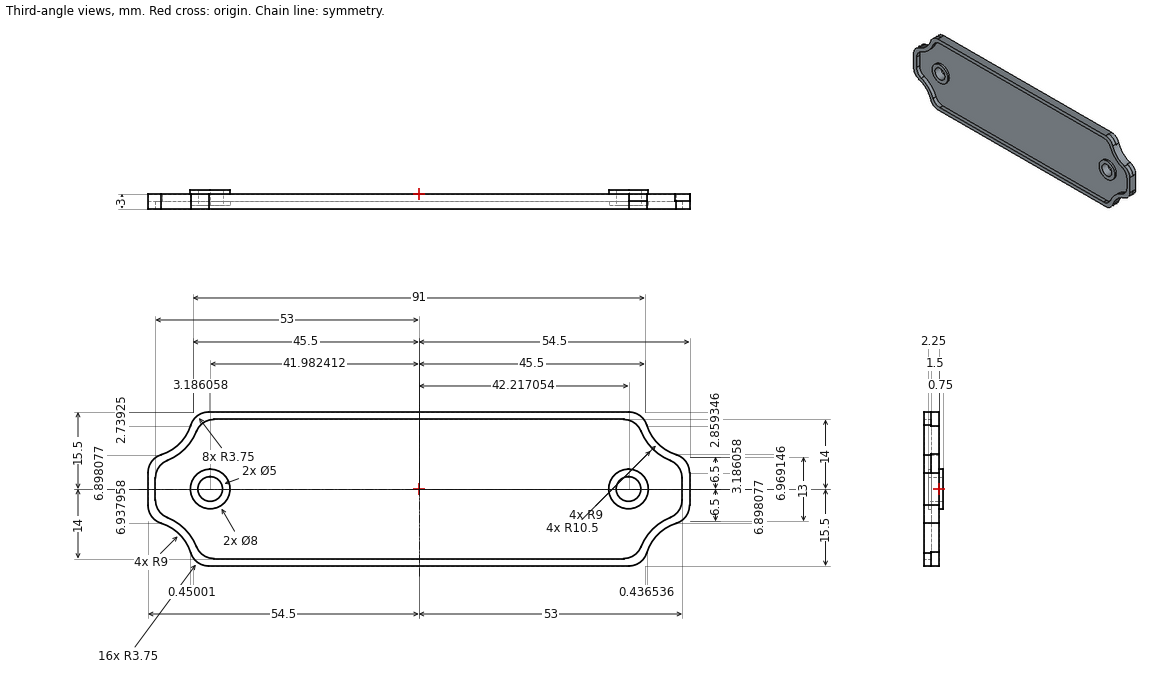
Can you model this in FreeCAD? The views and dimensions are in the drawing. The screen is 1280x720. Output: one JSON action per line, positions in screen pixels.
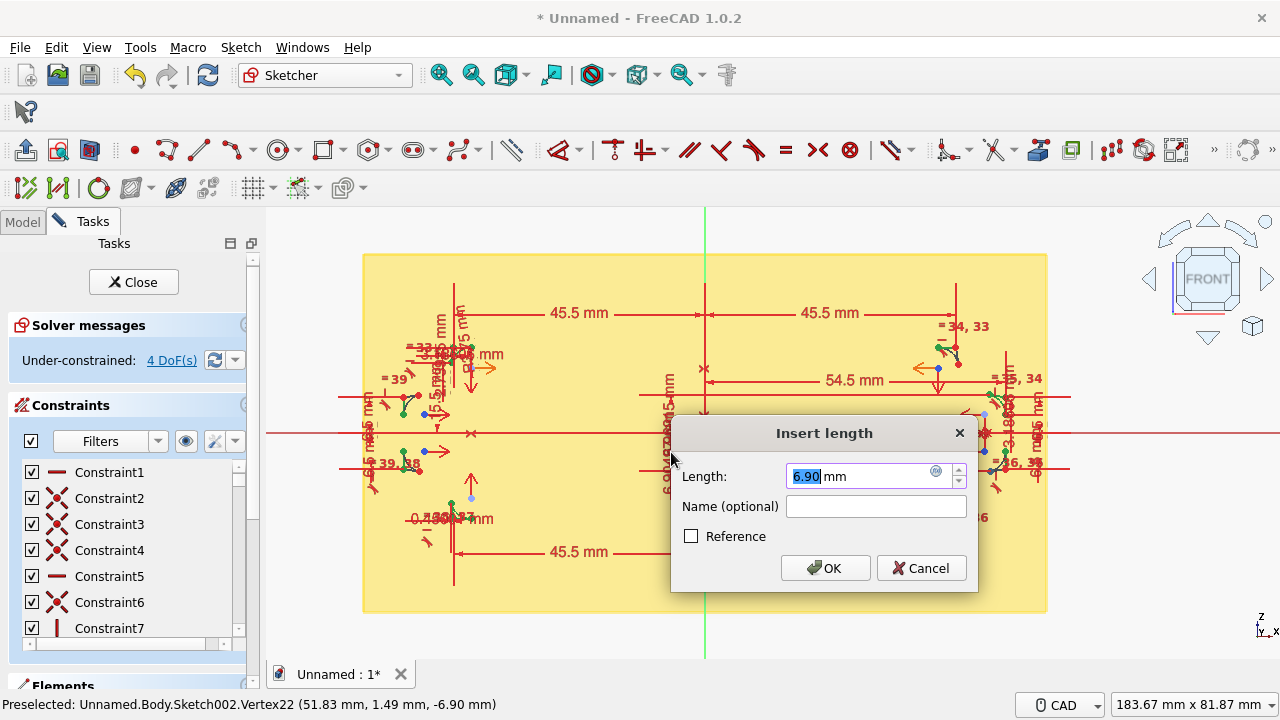
{"action": "type", "text": "6.898077"}
{"action": "key", "text": "Return"}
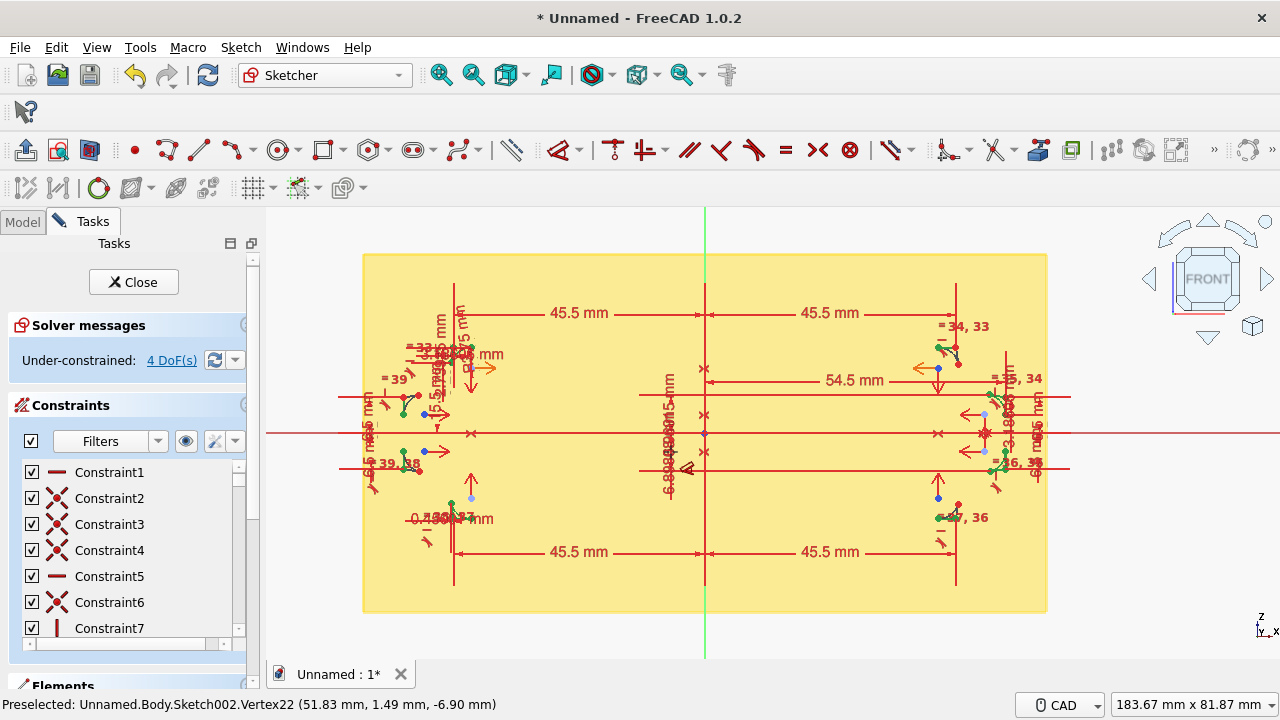
{"action": "left_click", "coordinate": [419, 472]}
{"action": "left_click", "coordinate": [763, 452]}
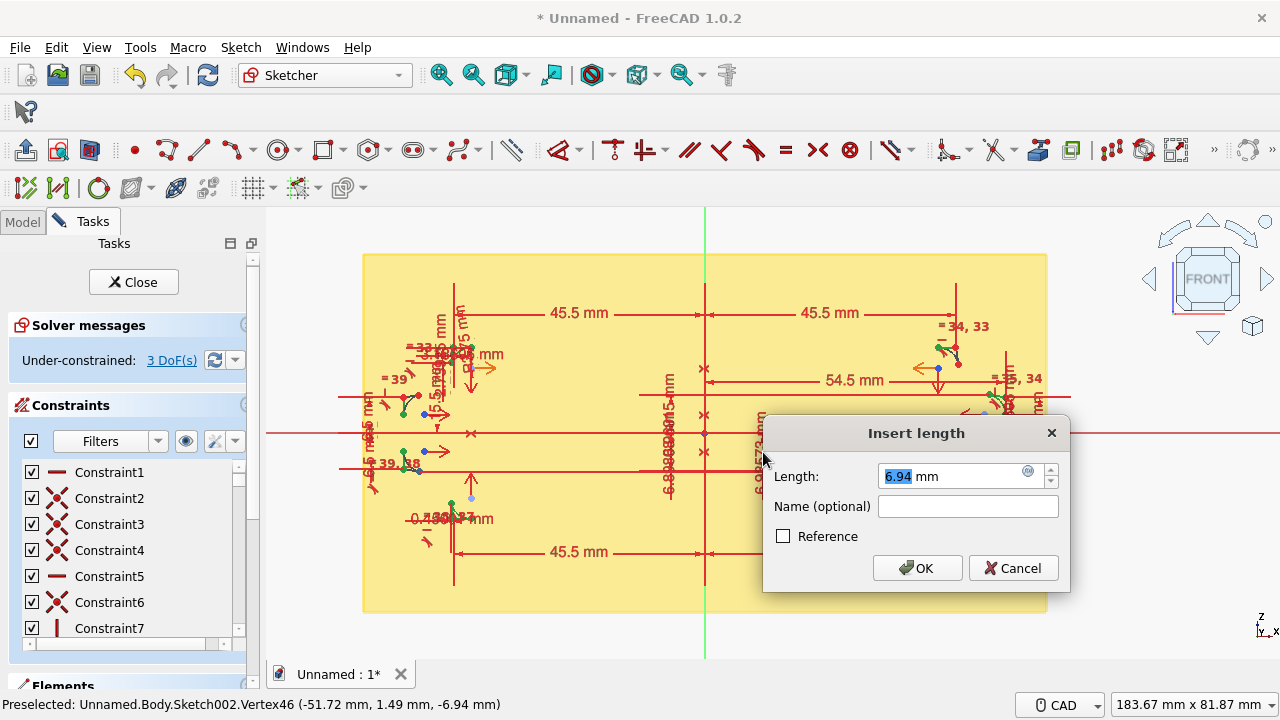
{"action": "type", "text": "6.937958"}
{"action": "key", "text": "Return"}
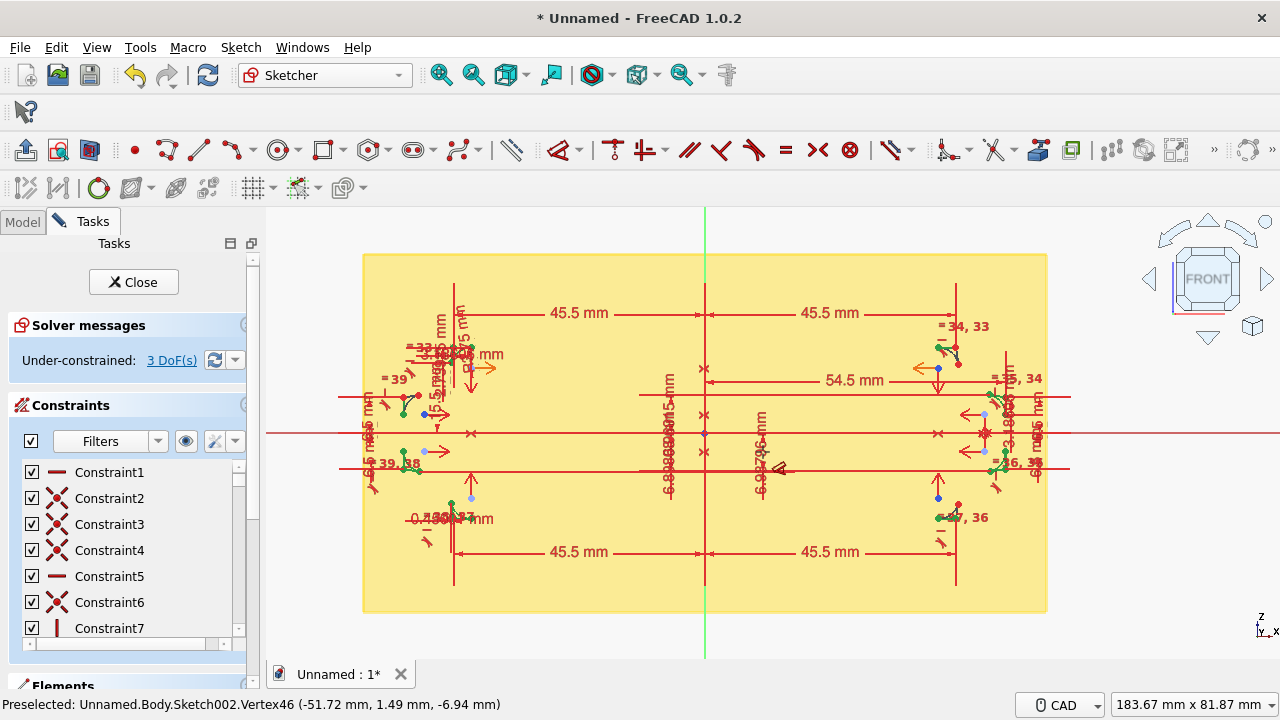
{"action": "left_click", "coordinate": [418, 395]}
{"action": "left_click", "coordinate": [763, 414]}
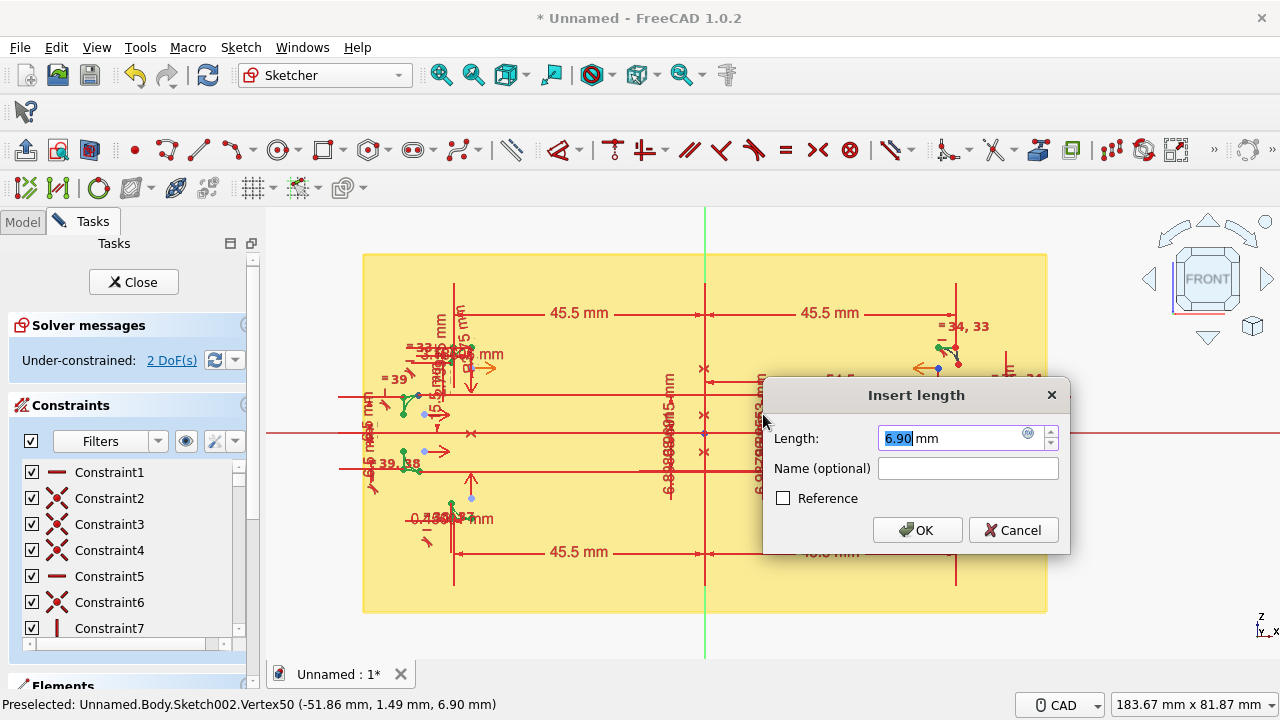
{"action": "type", "text": "6.898077"}
{"action": "key", "text": "Return"}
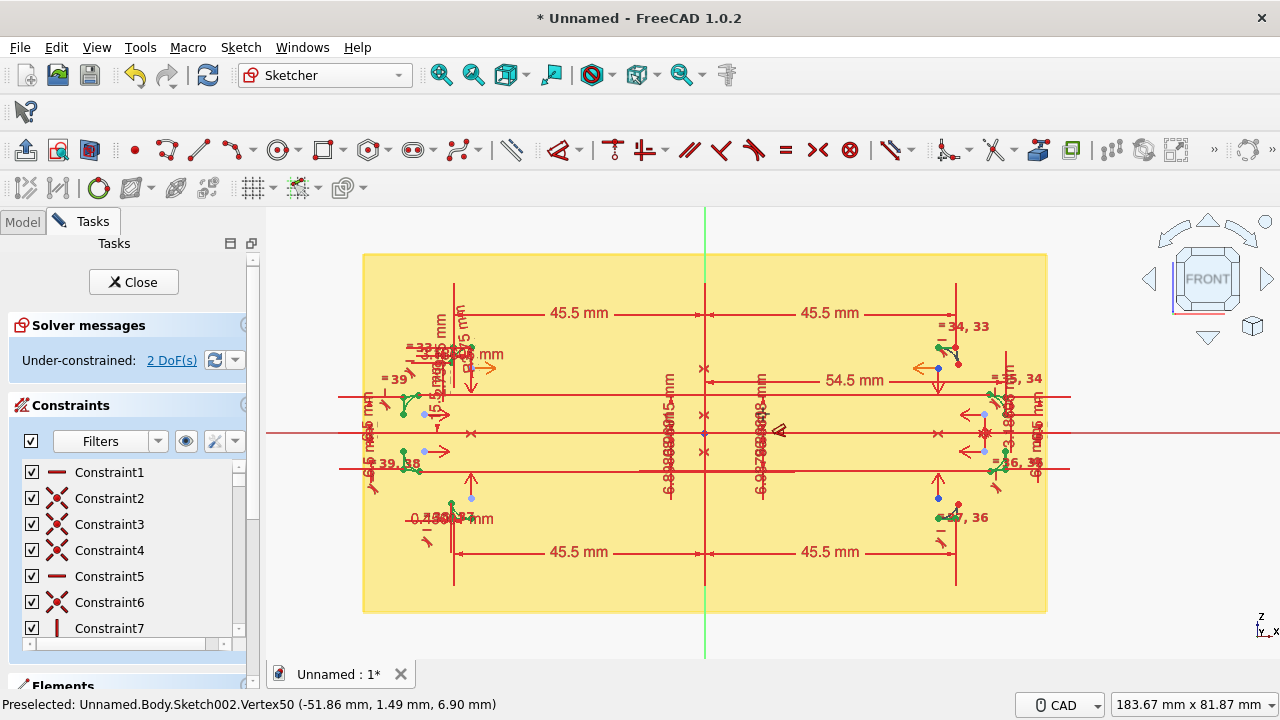
{"action": "scroll", "coordinate": [957, 353], "scroll_direction": "up", "scroll_amount": 7}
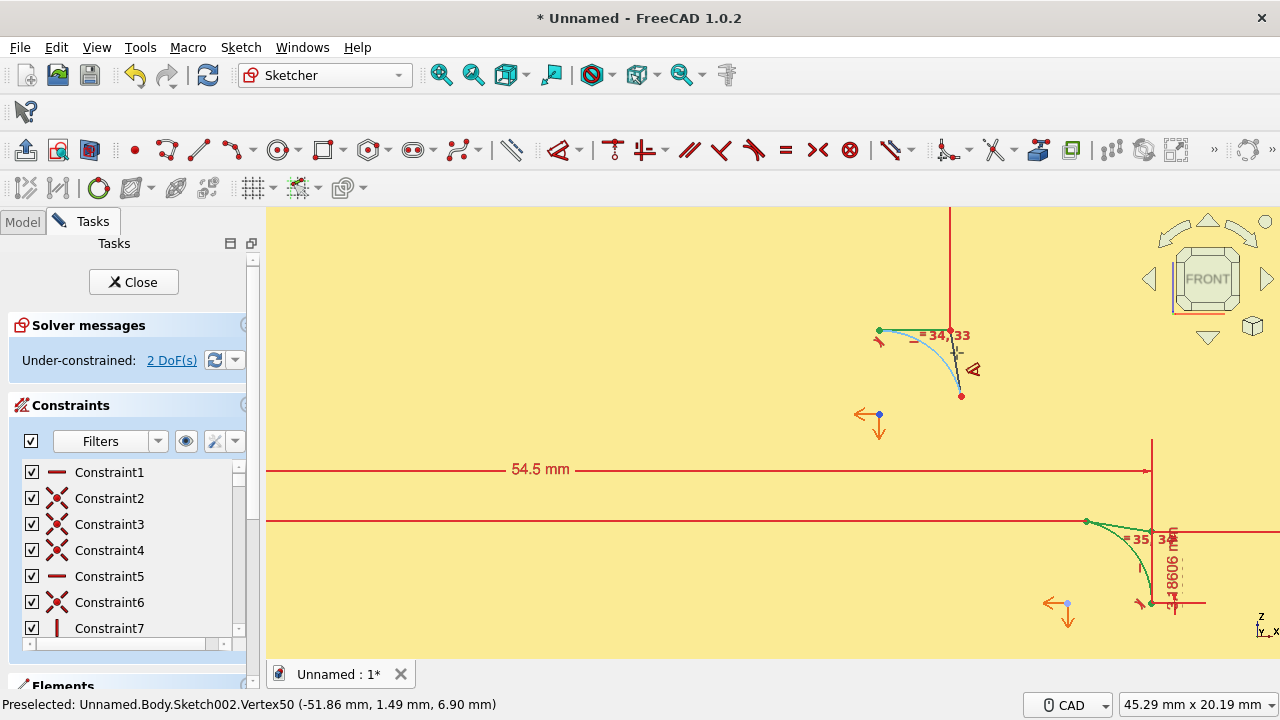
{"action": "left_click", "coordinate": [954, 350]}
{"action": "left_click", "coordinate": [995, 364]}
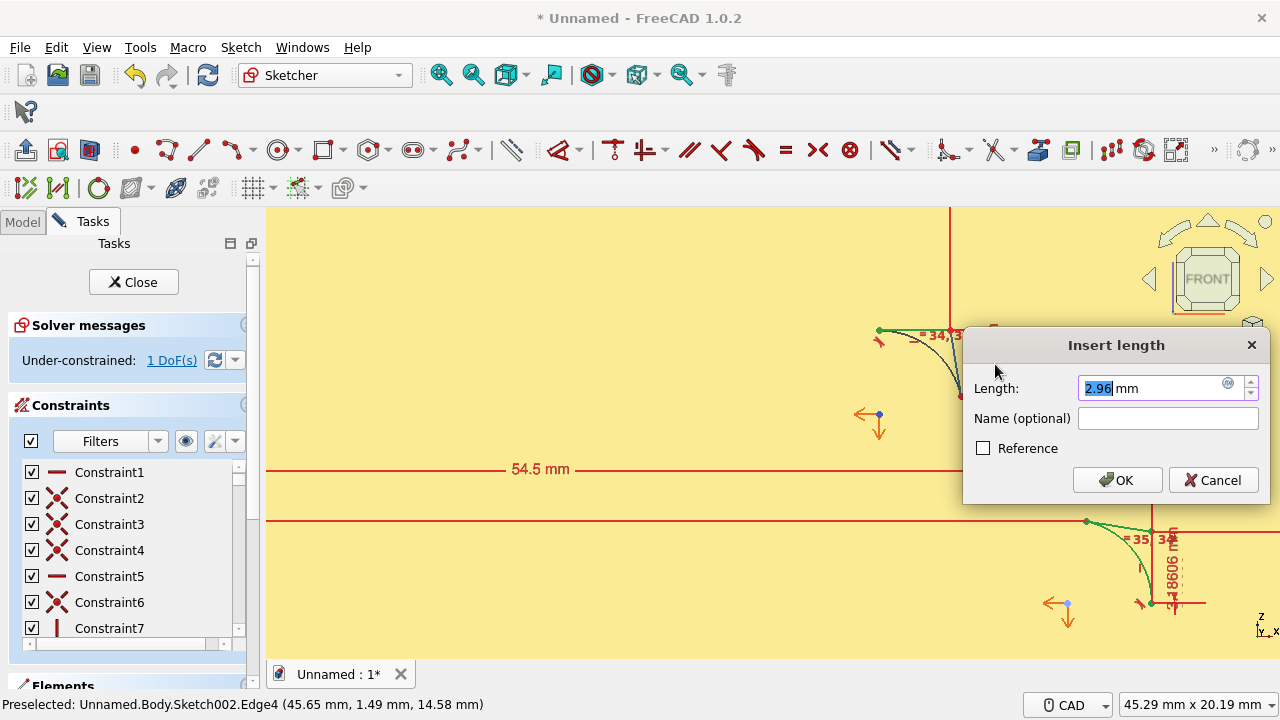
{"action": "type", "text": "2.859346"}
{"action": "key", "text": "Return"}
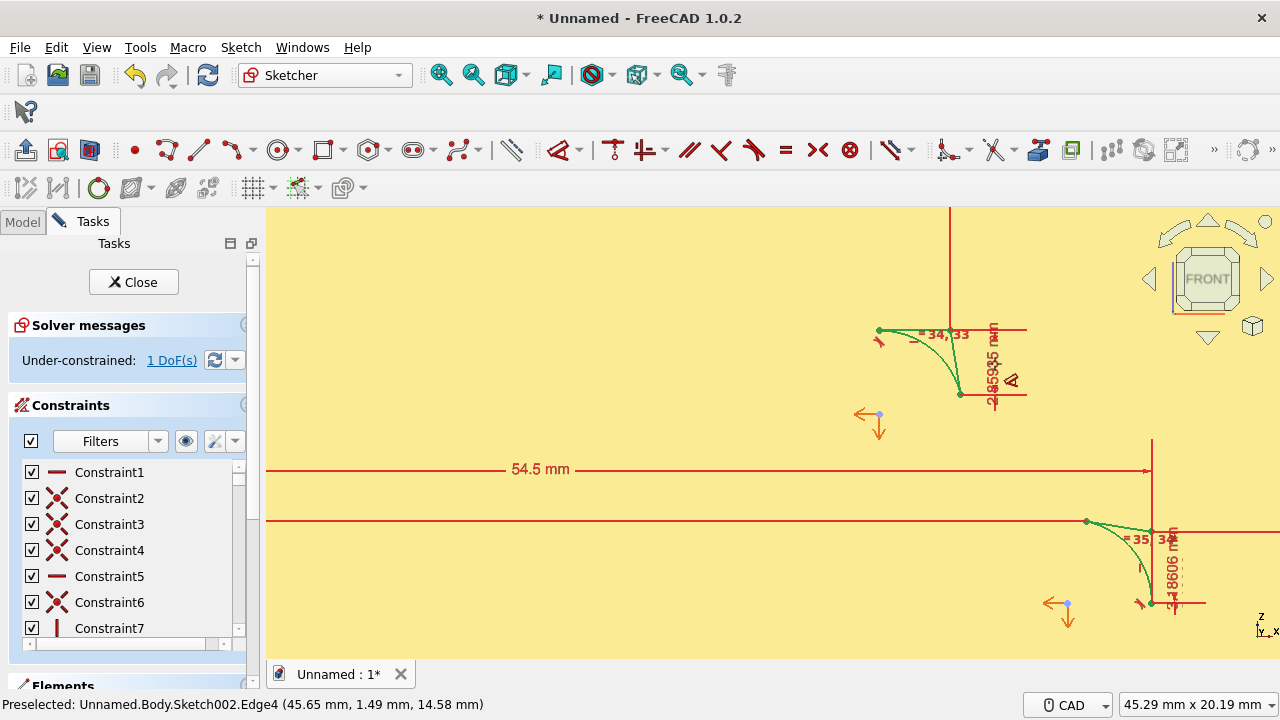
{"action": "scroll", "coordinate": [957, 353], "scroll_direction": "down", "scroll_amount": 7}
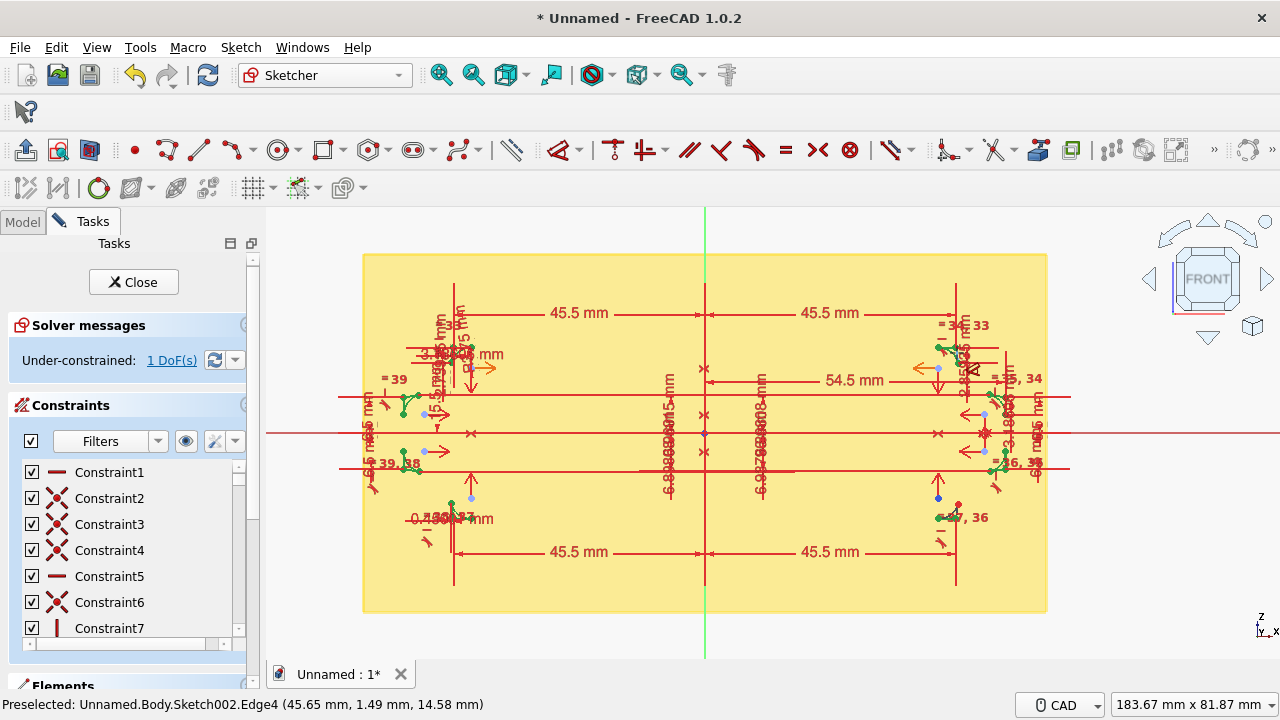
{"action": "scroll", "coordinate": [957, 515], "scroll_direction": "up", "scroll_amount": 15}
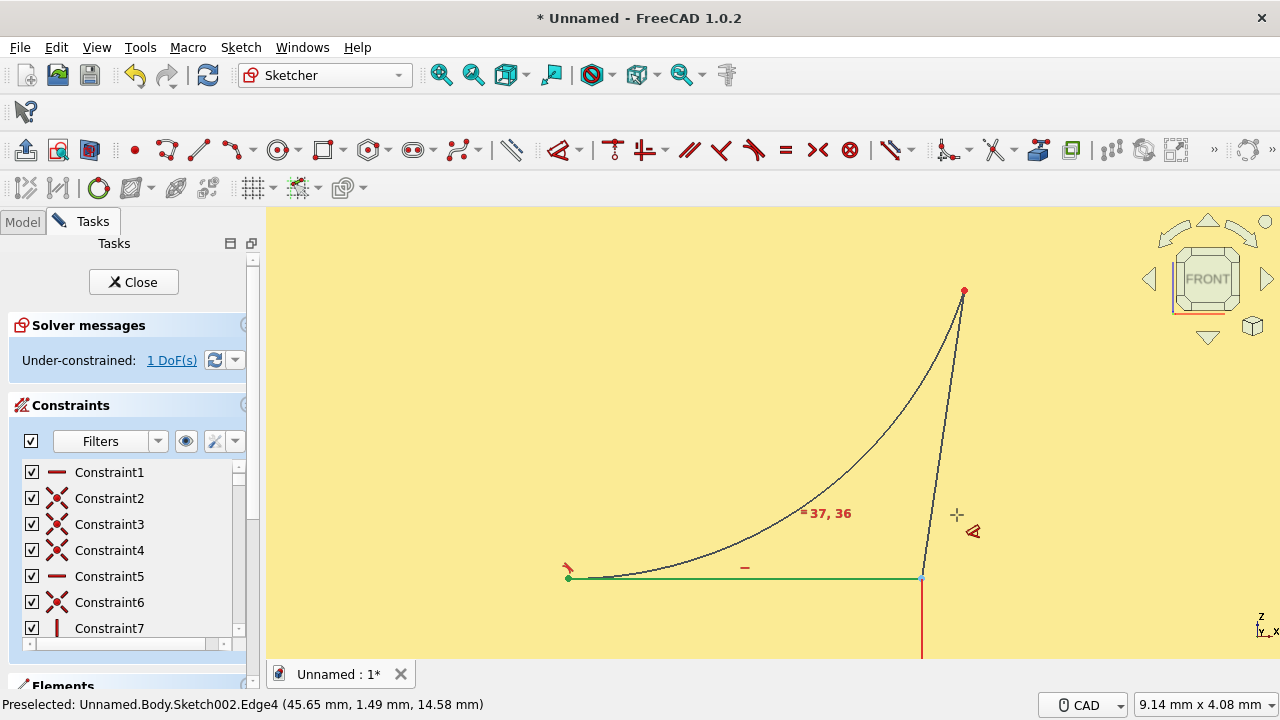
{"action": "left_click", "coordinate": [935, 492]}
{"action": "left_click", "coordinate": [943, 613]}